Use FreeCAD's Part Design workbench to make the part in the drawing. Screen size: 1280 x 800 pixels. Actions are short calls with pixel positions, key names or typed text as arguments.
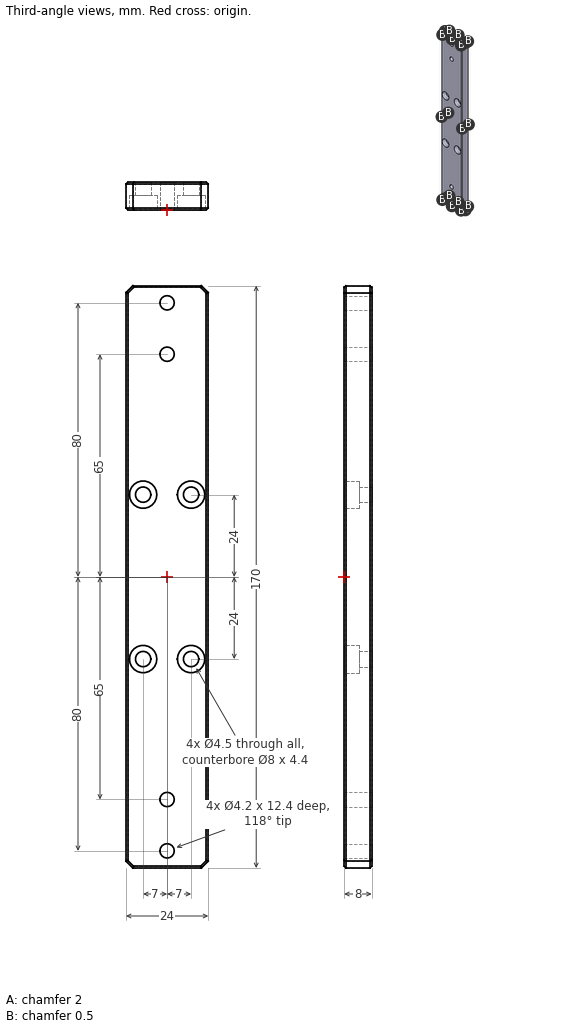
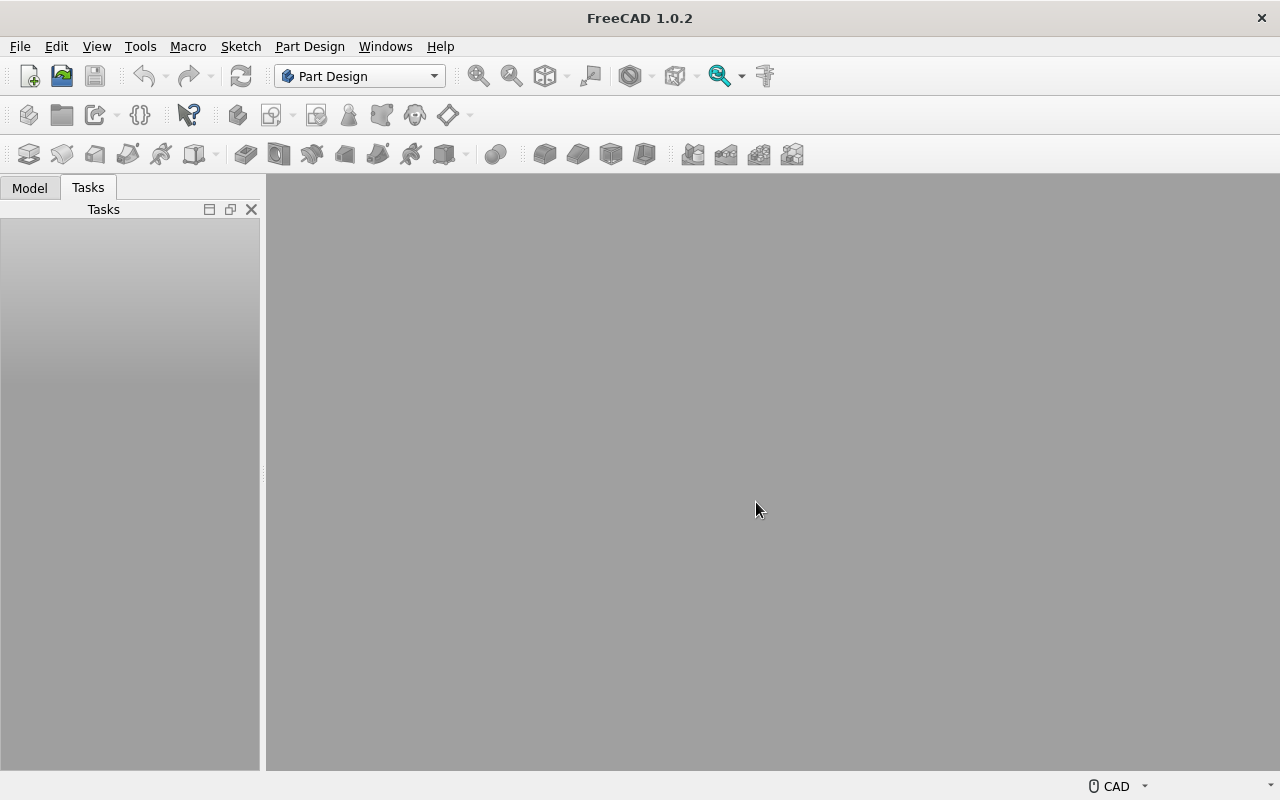
click(29, 76)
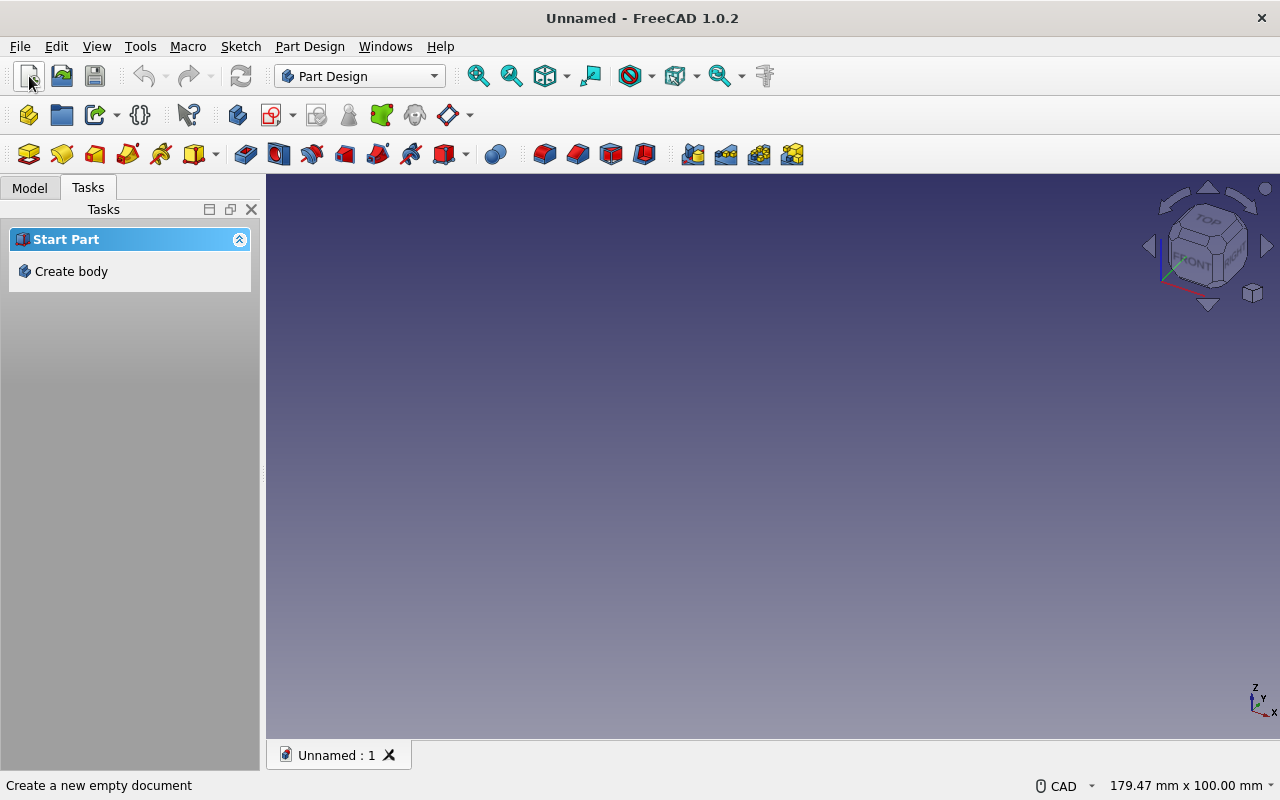
click(270, 116)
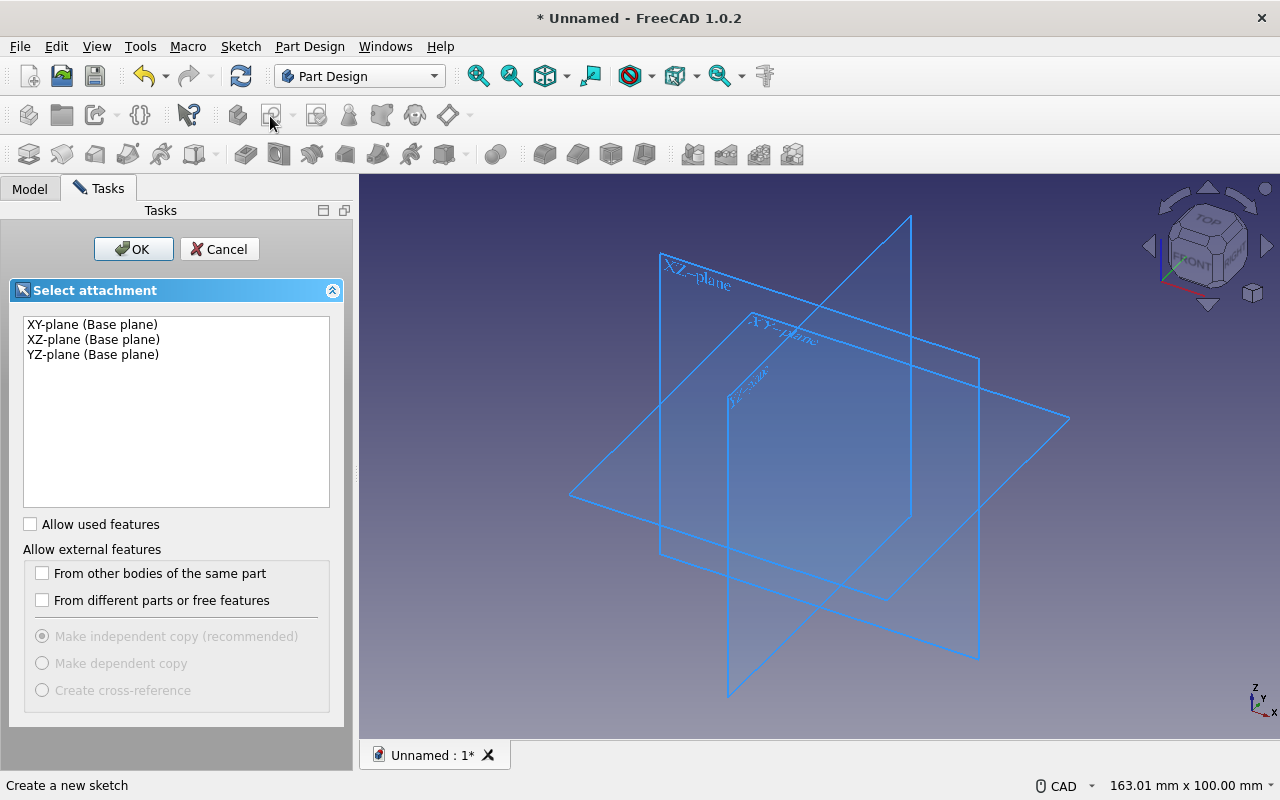
click(84, 340)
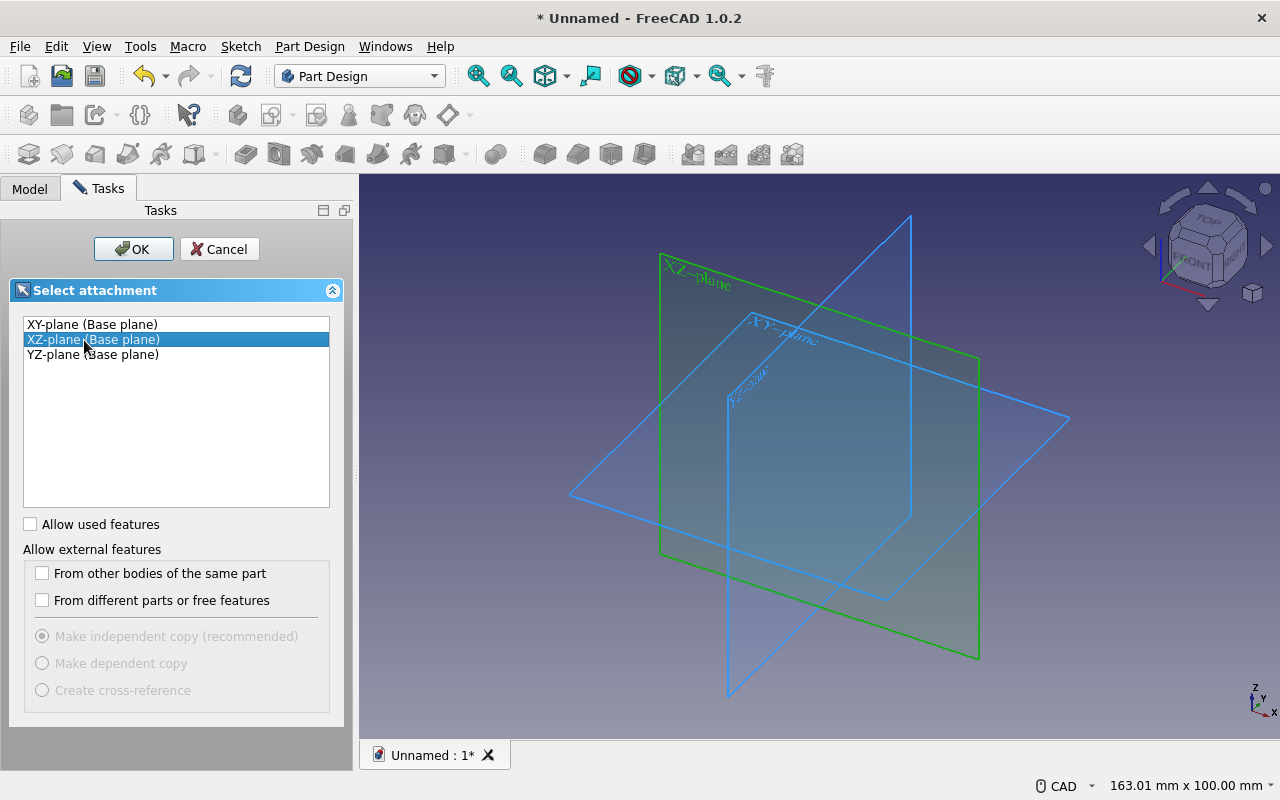
click(134, 249)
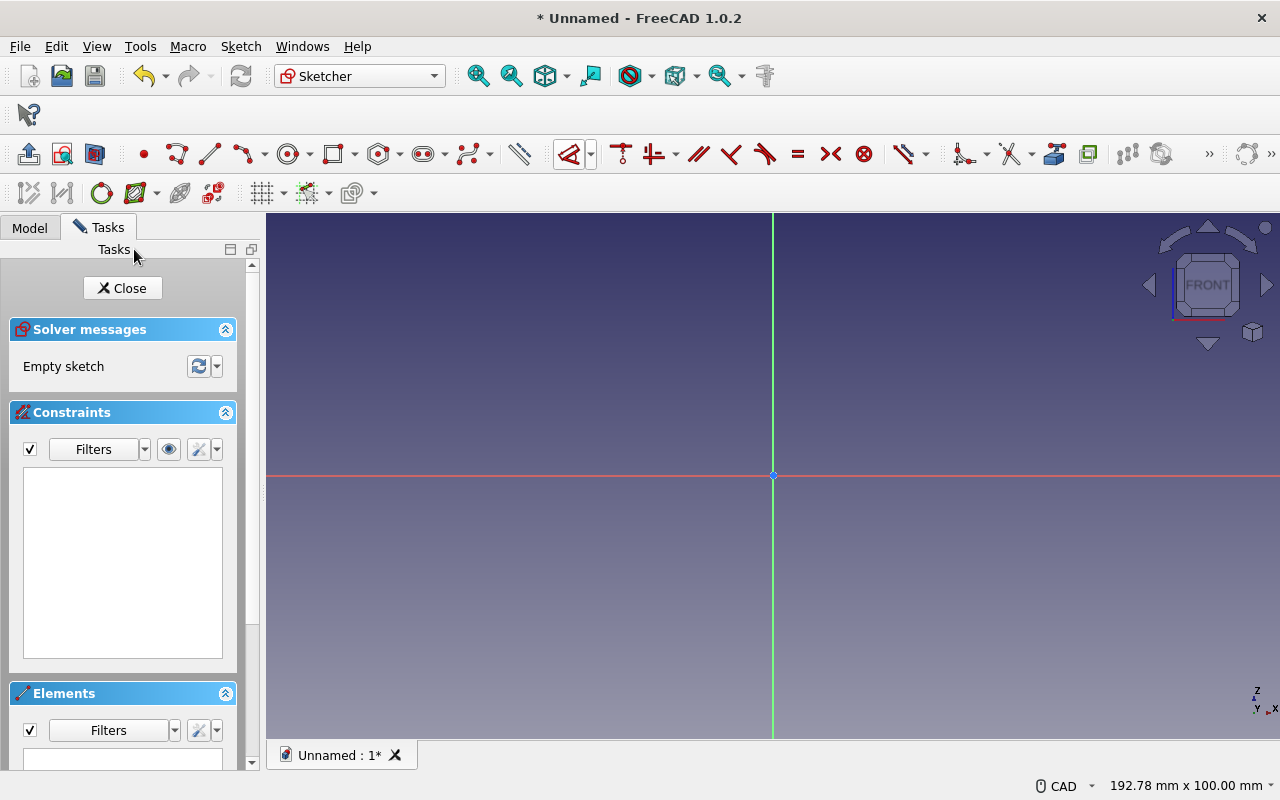
scroll(665, 476, down, 5)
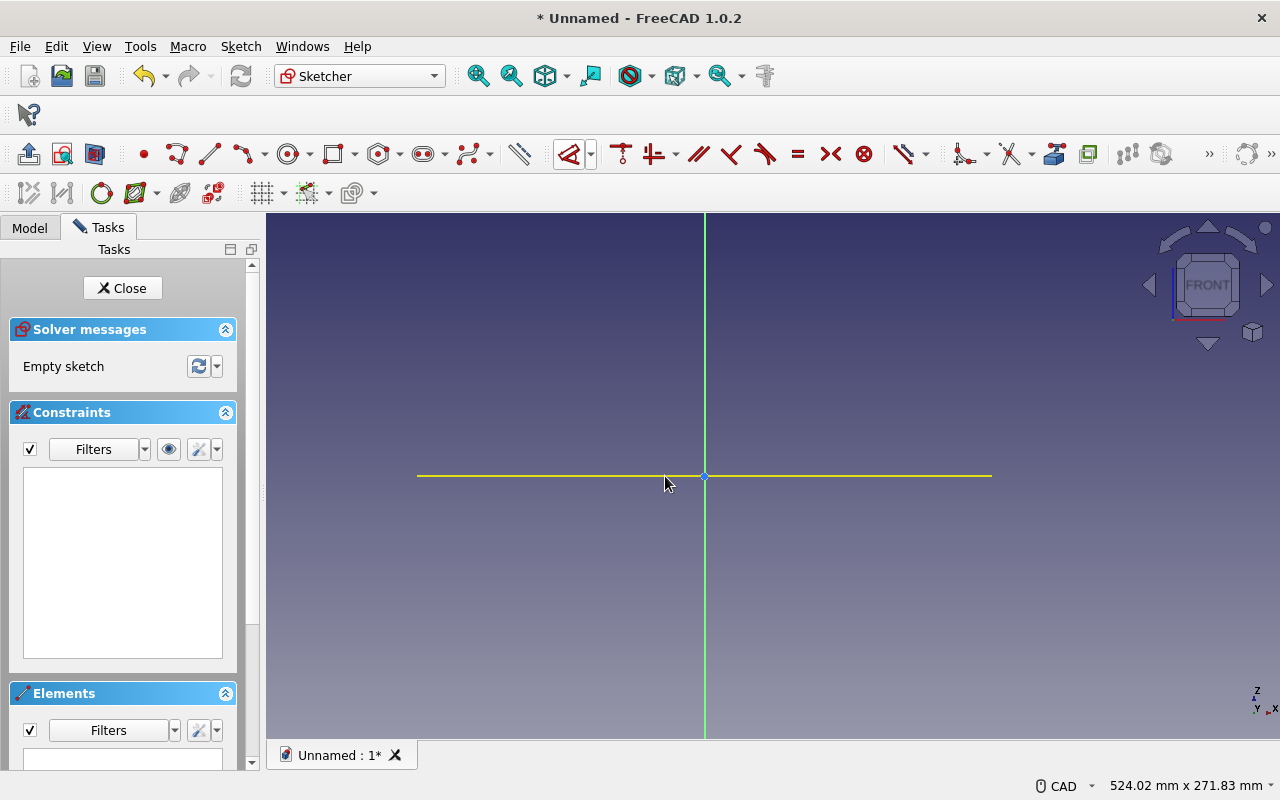
key(g)
key(v)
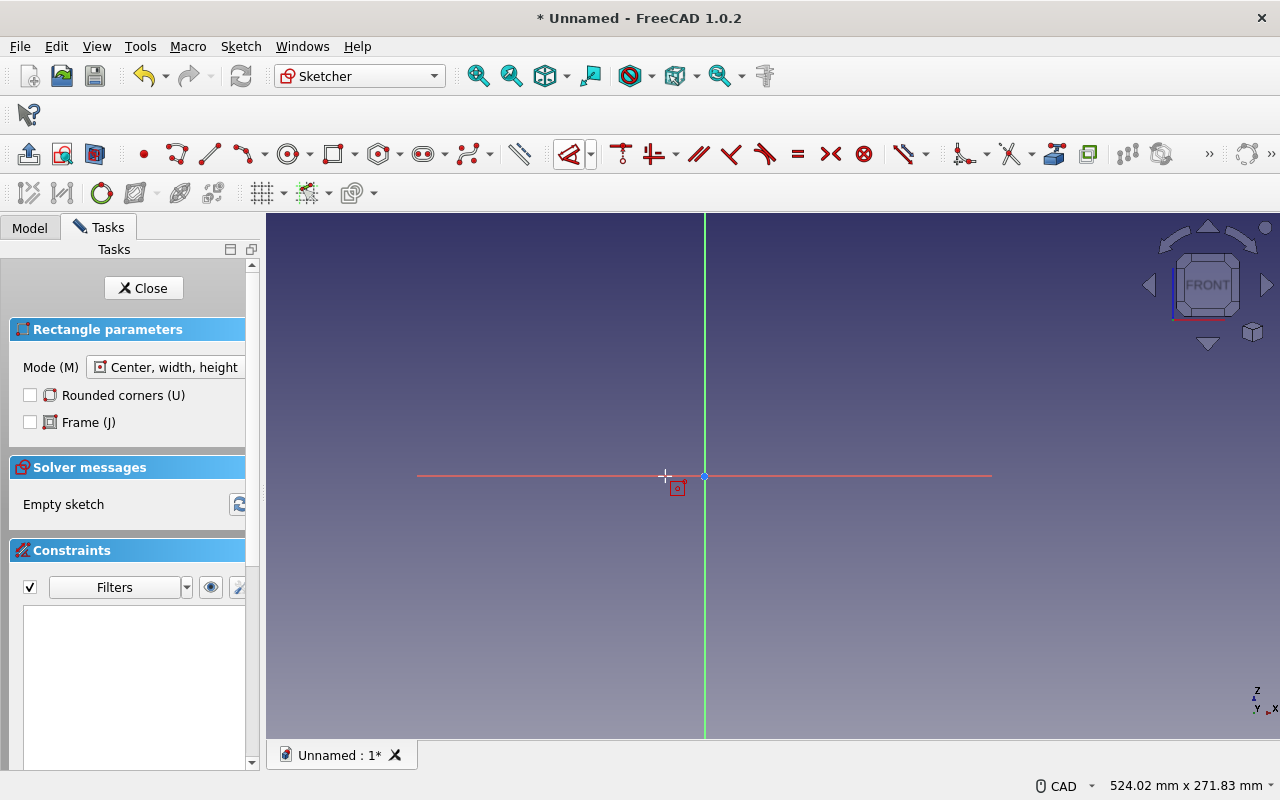
click(705, 476)
move(728, 312)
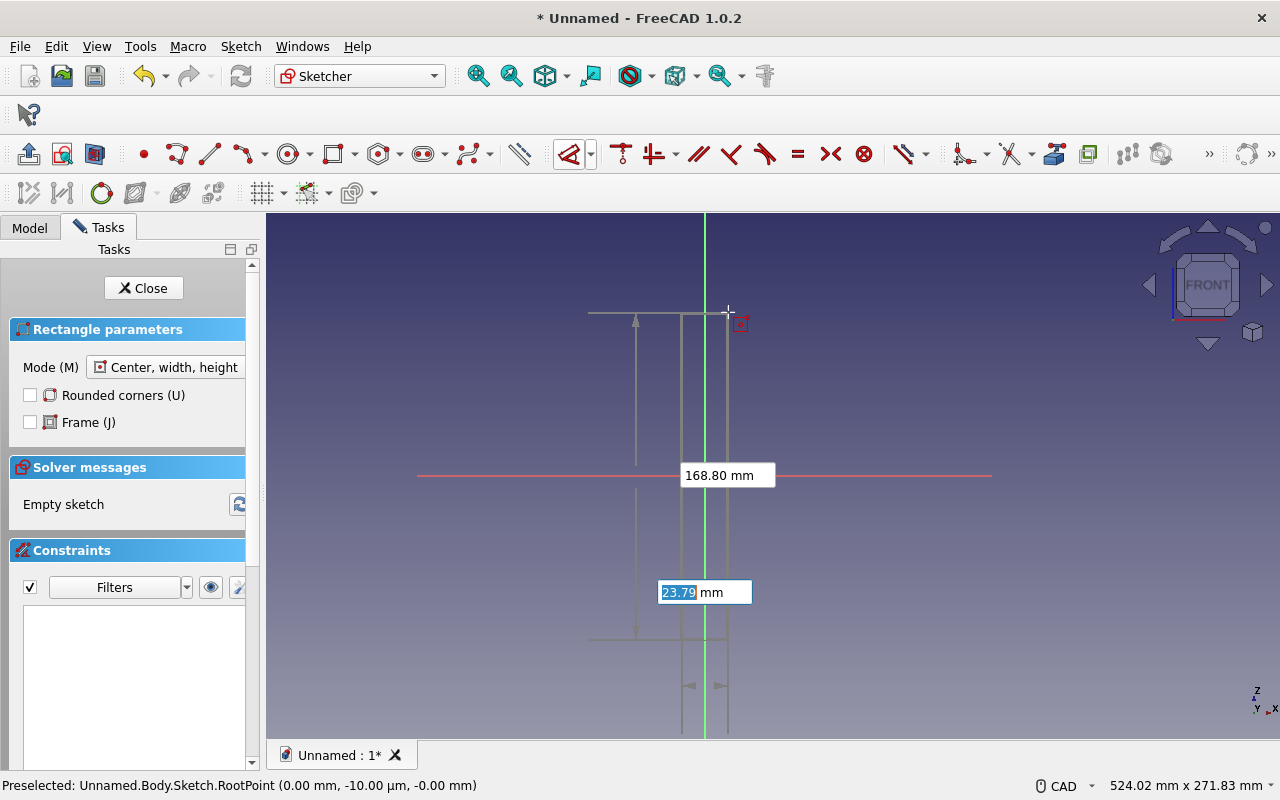
text(24)
key(Tab)
text(170)
key(Return)
key(Escape)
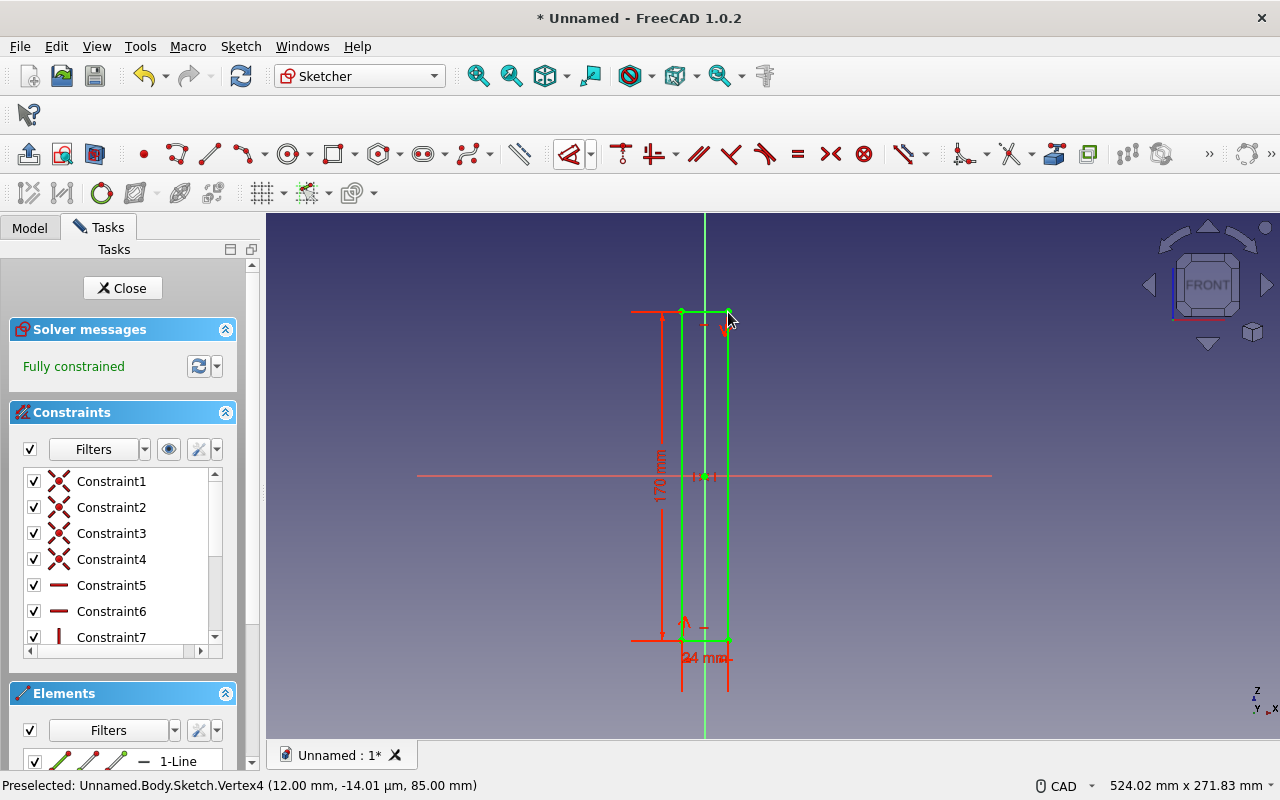
click(123, 288)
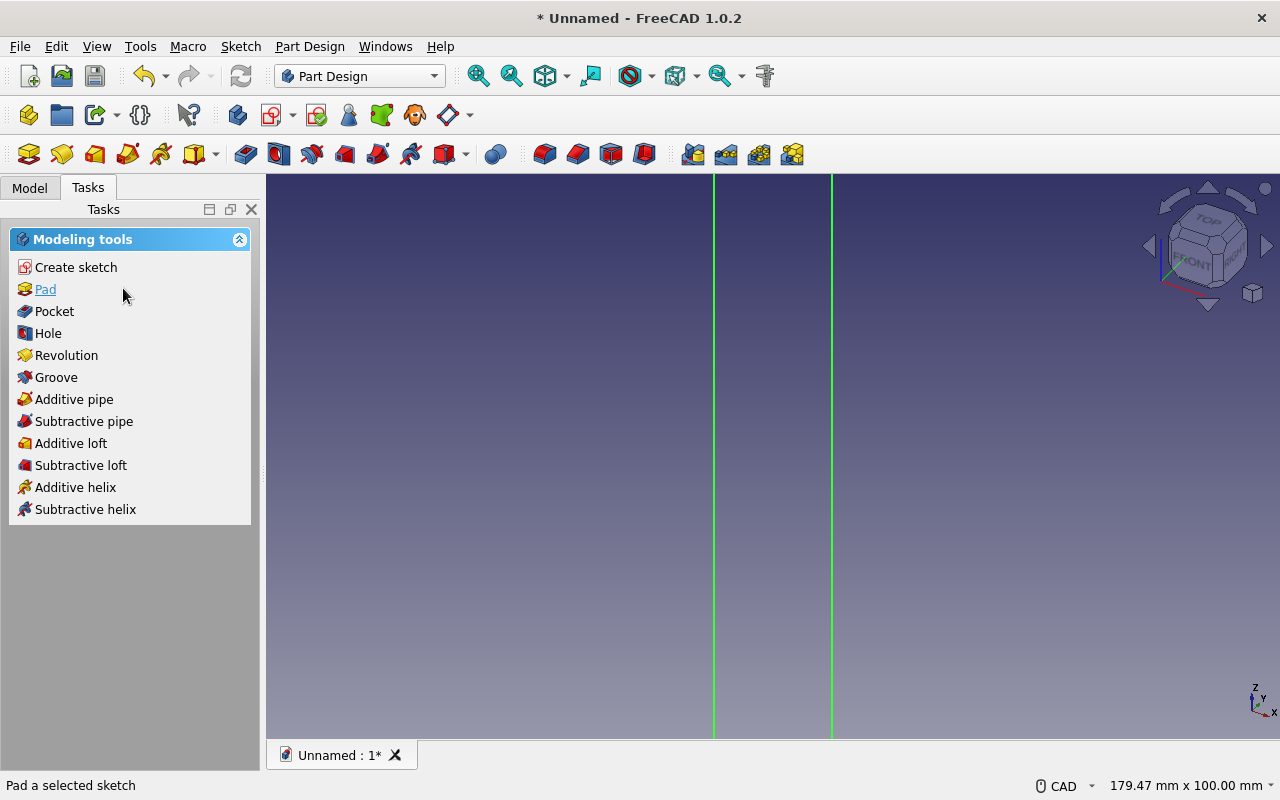
click(29, 154)